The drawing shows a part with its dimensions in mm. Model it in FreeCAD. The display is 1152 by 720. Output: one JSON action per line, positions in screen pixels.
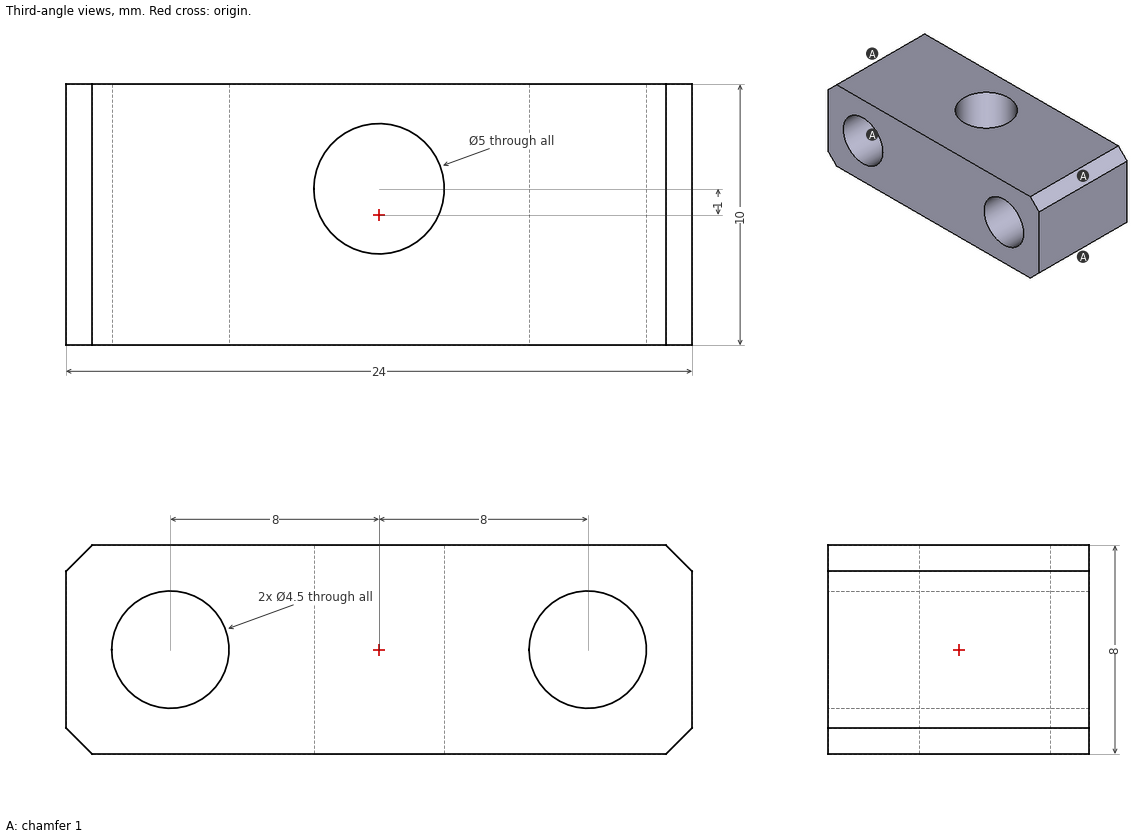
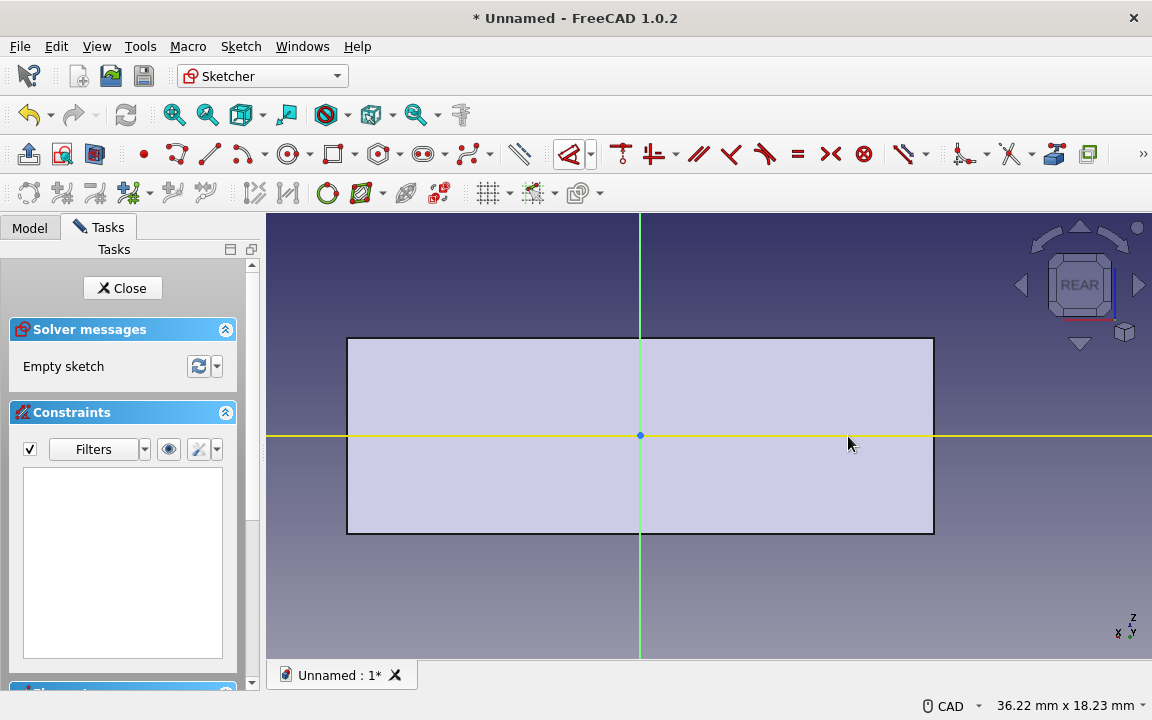
{"action": "left_click", "coordinate": [288, 154]}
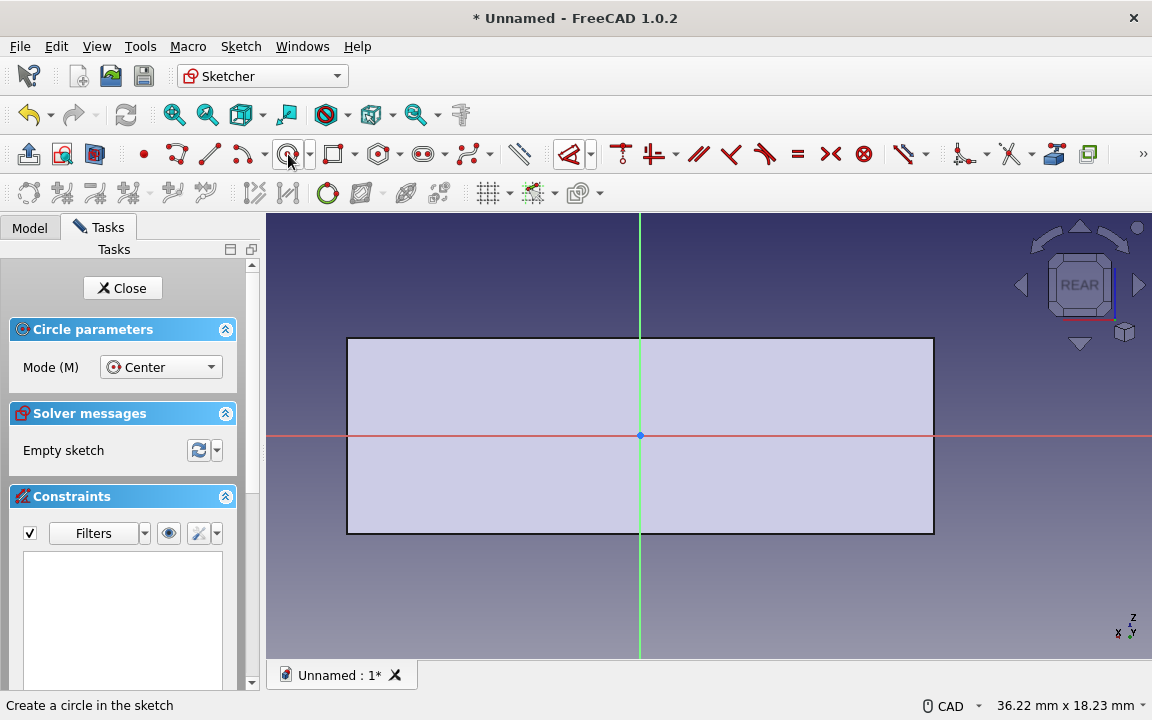
{"action": "left_click", "coordinate": [836, 436]}
{"action": "left_click", "coordinate": [875, 397]}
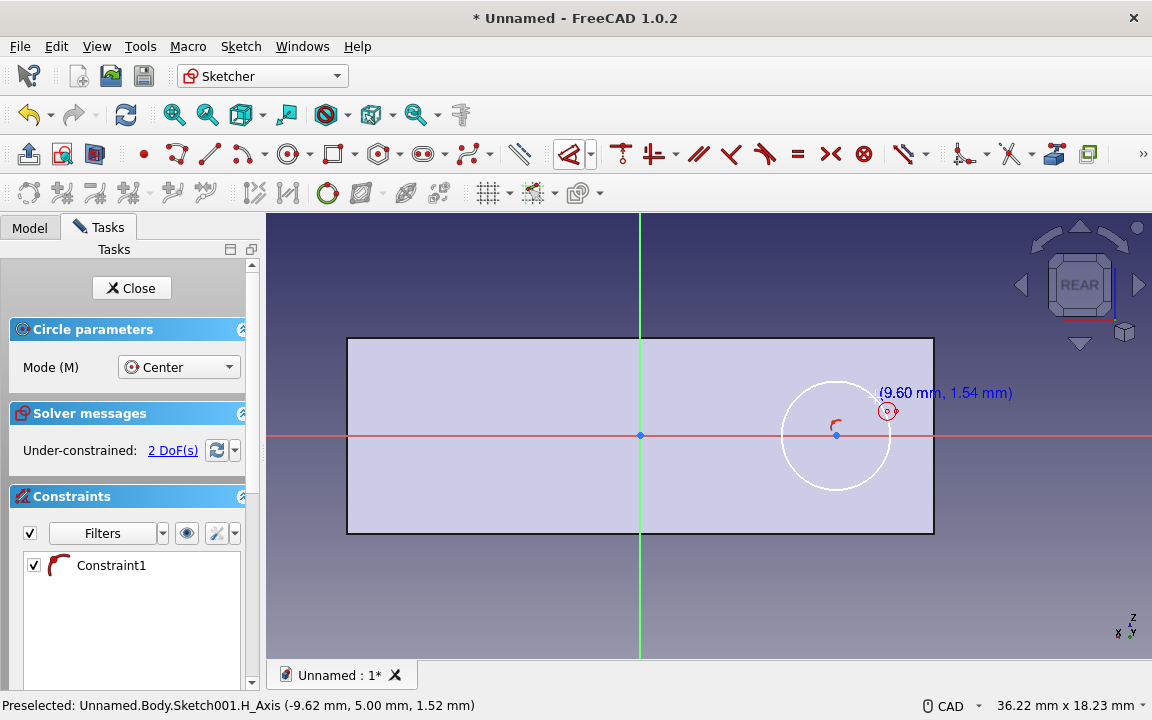
{"action": "left_click", "coordinate": [445, 436]}
{"action": "left_click", "coordinate": [484, 397]}
{"action": "key", "text": "Escape"}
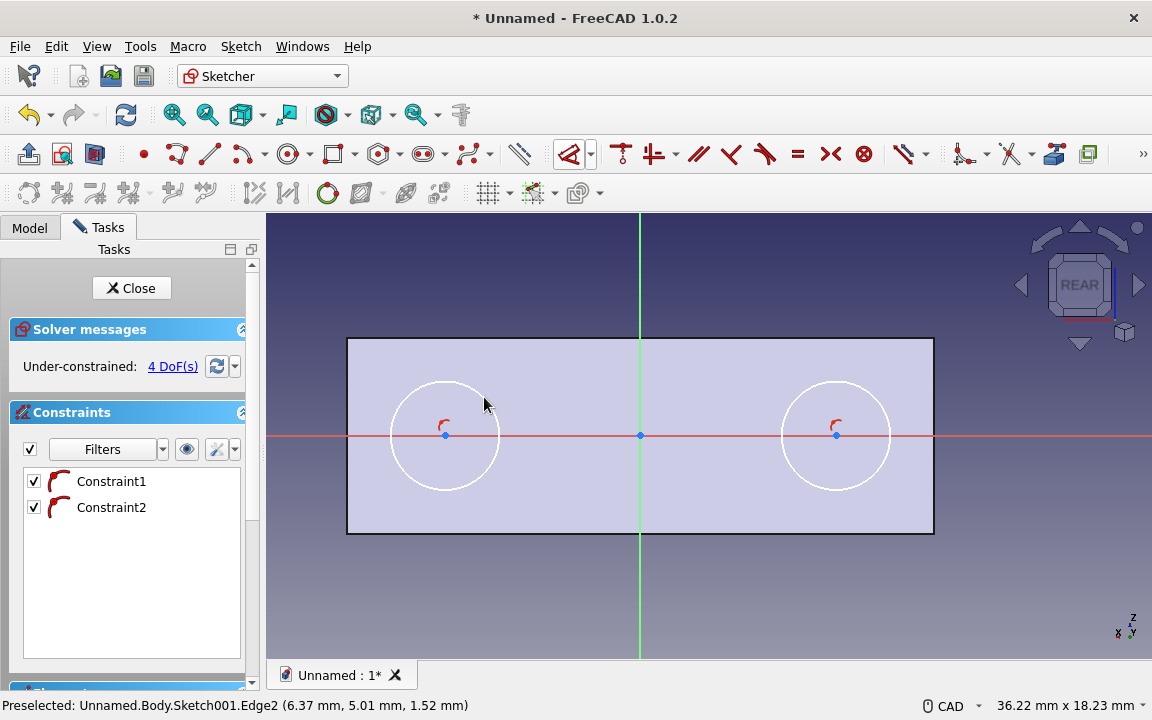
{"action": "left_click", "coordinate": [874, 397]}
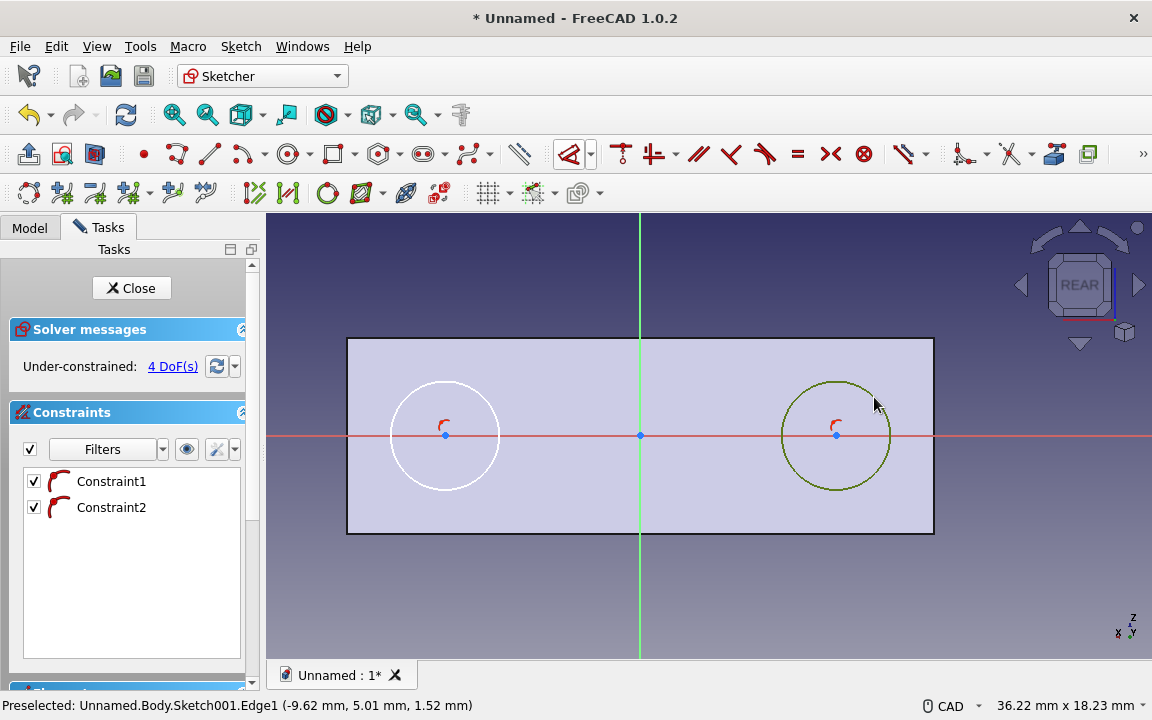
{"action": "left_click", "coordinate": [483, 397]}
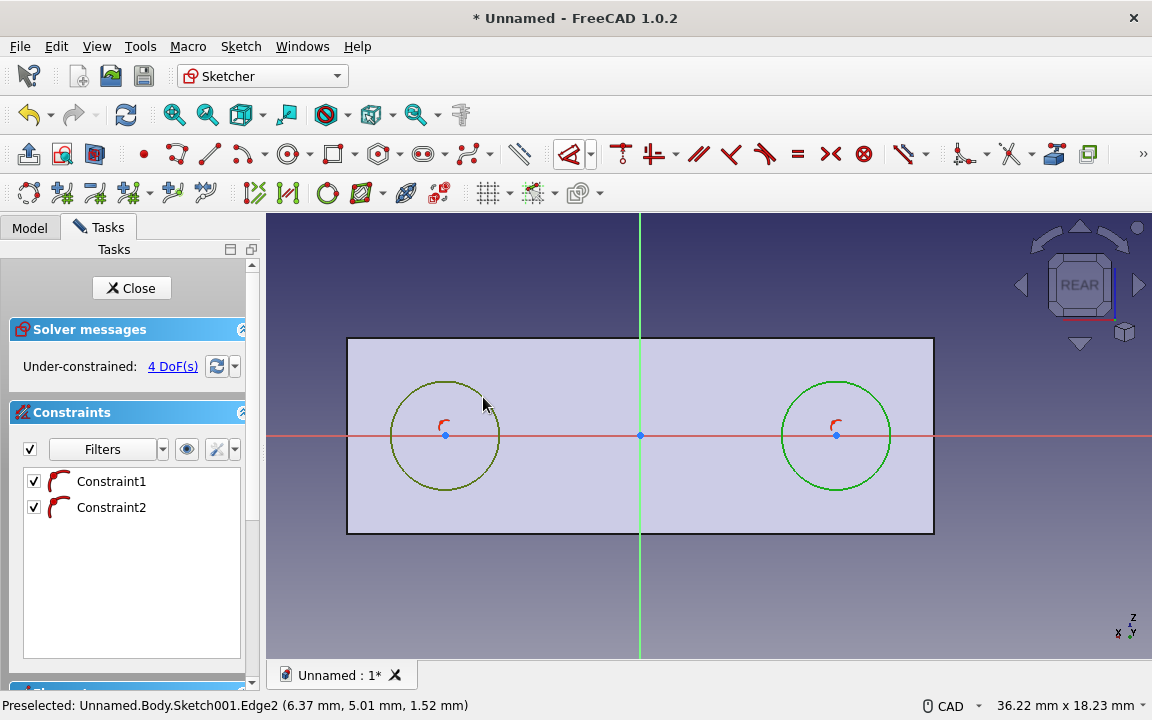
{"action": "left_click", "coordinate": [798, 154]}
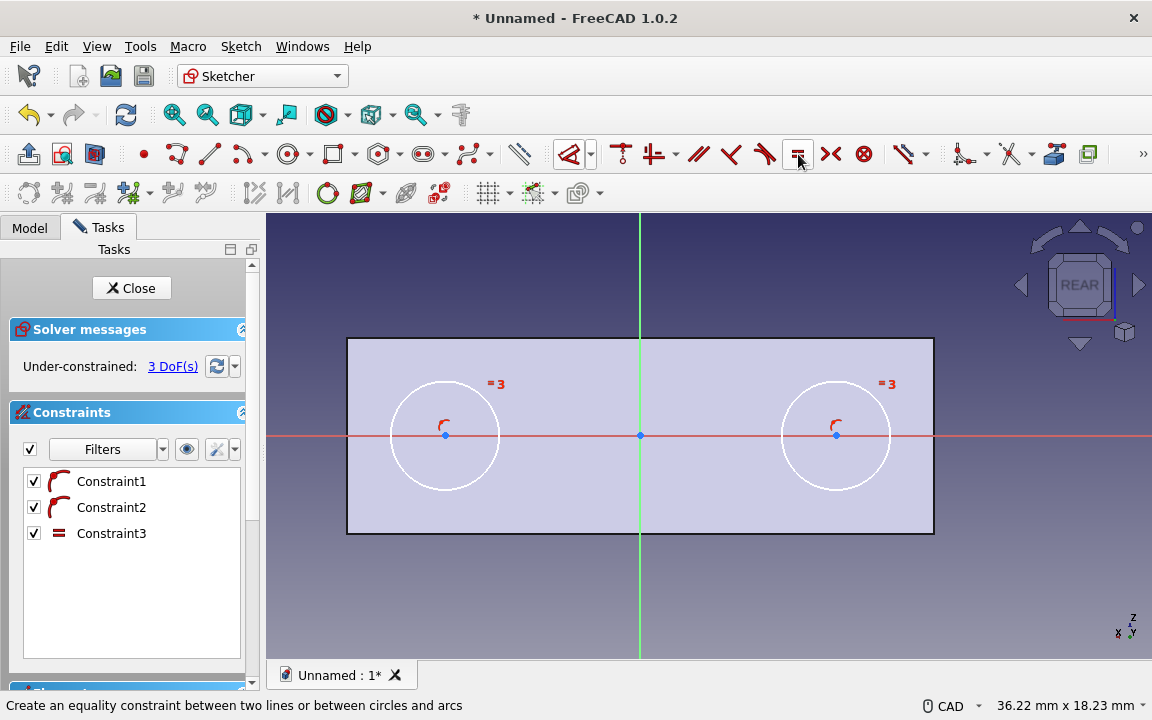
{"action": "left_click", "coordinate": [874, 397]}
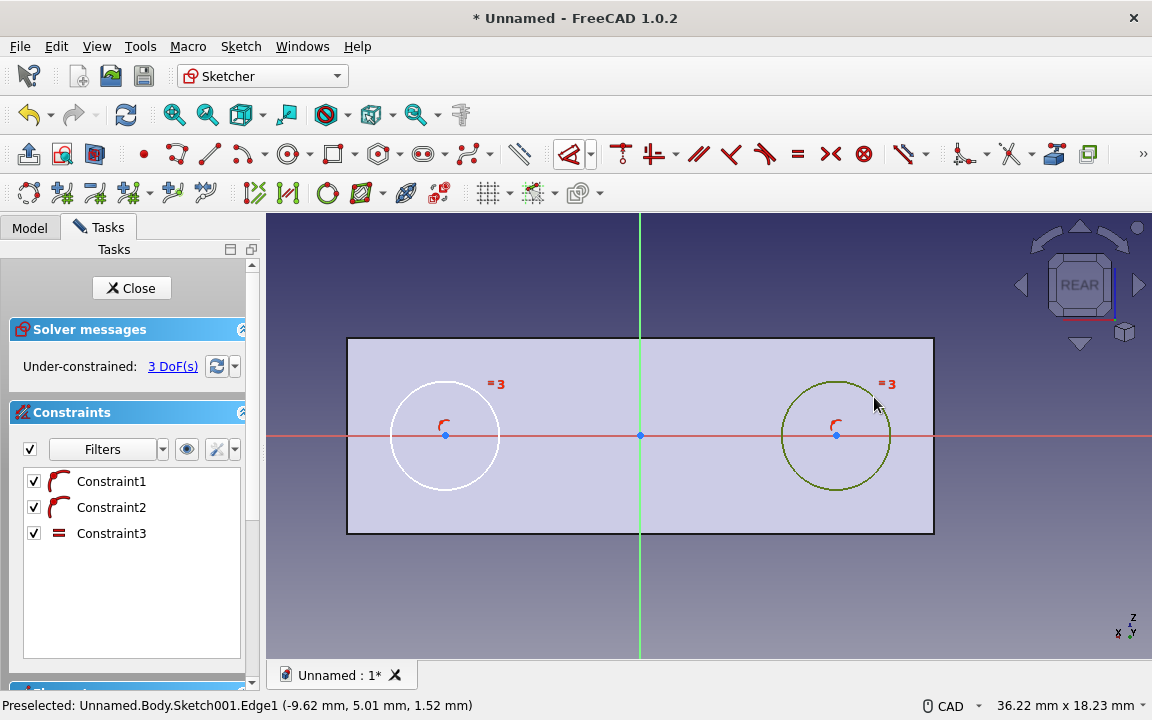
{"action": "key", "text": "k o"}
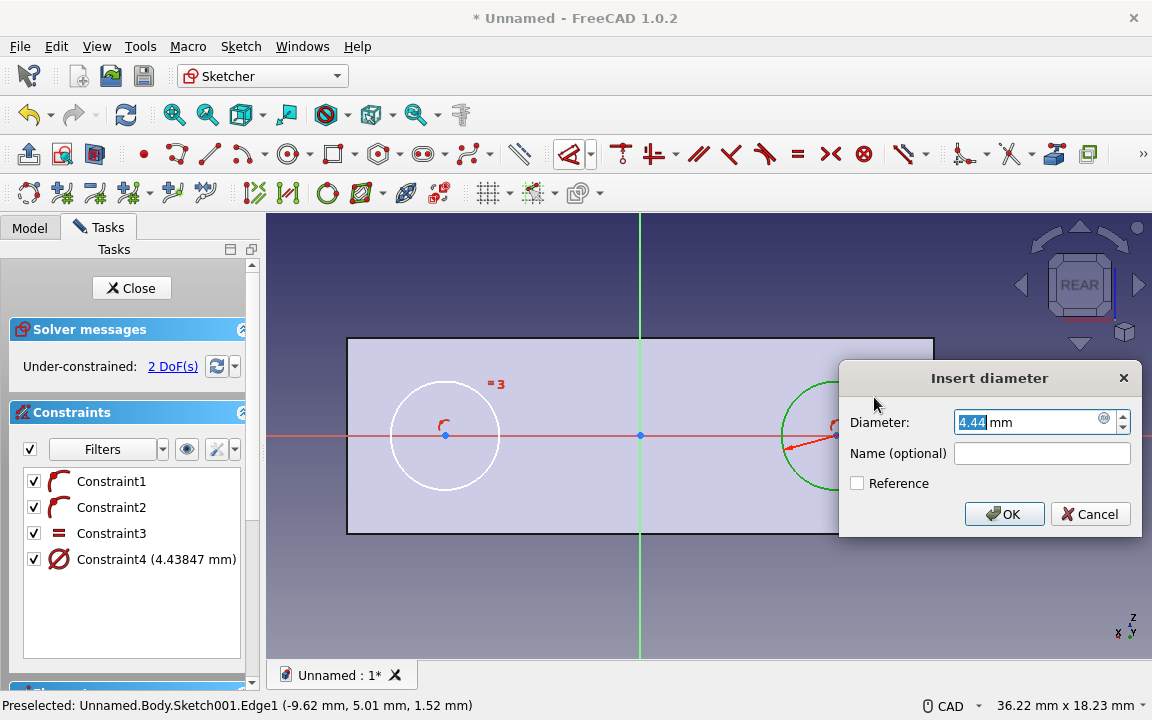
{"action": "type", "text": "4.5"}
{"action": "key", "text": "Return"}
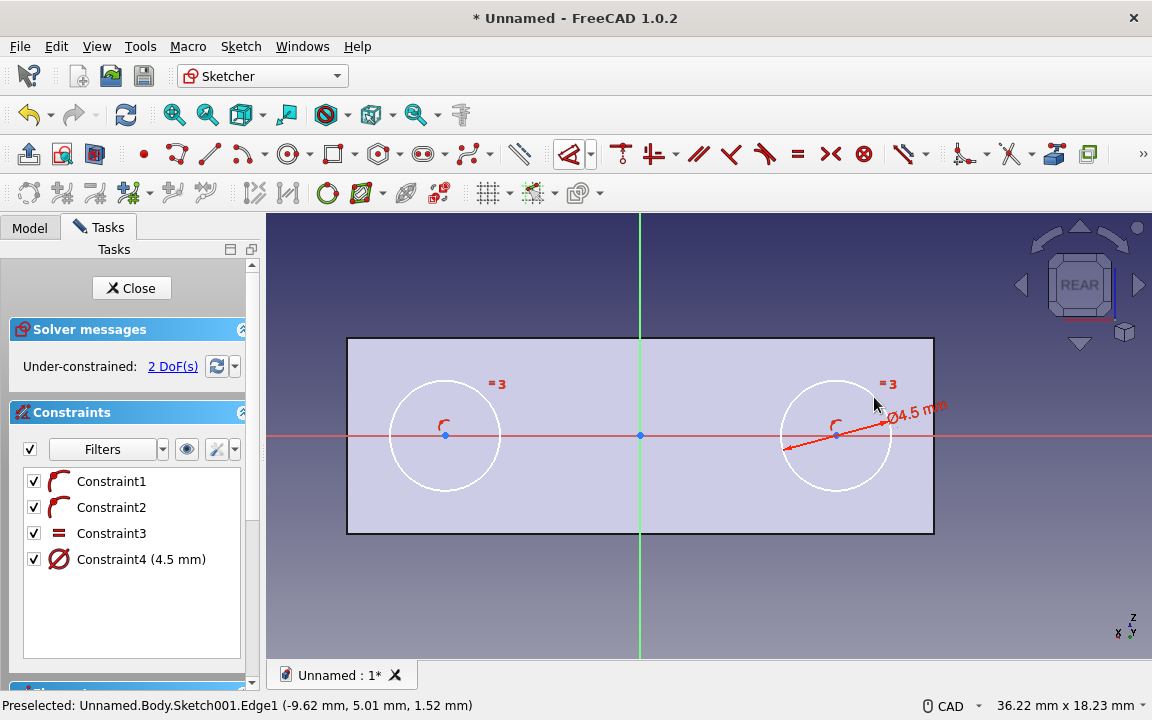
{"action": "left_click", "coordinate": [836, 436]}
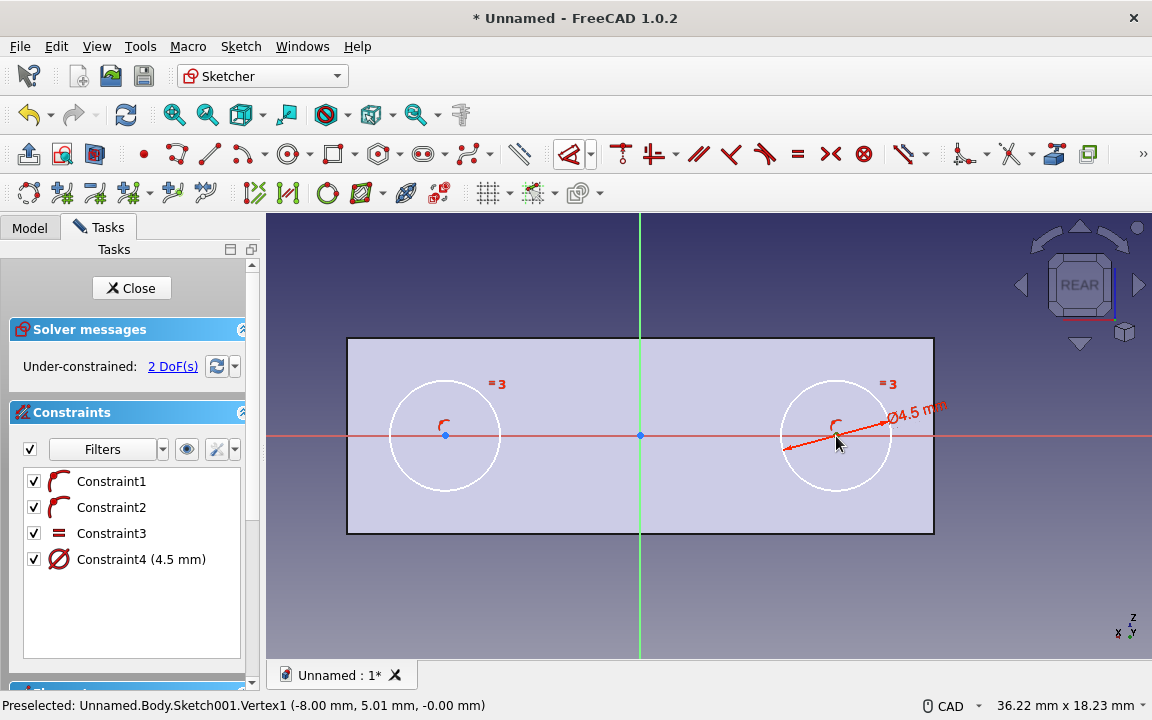
{"action": "key", "text": "l"}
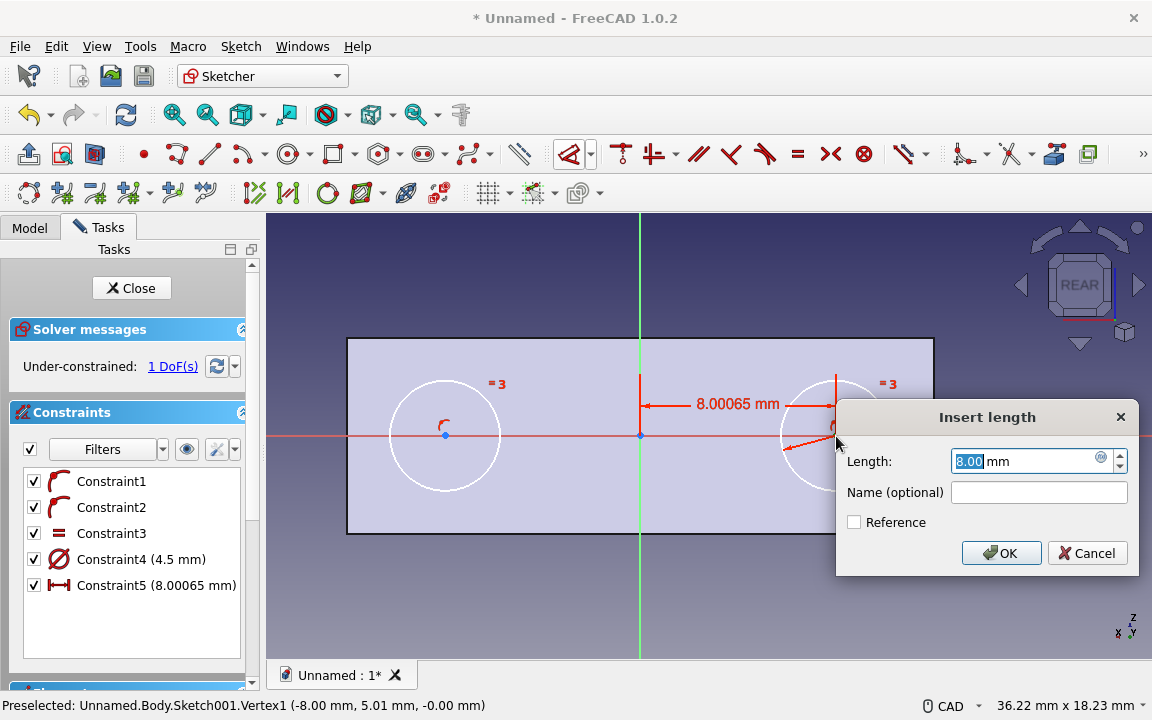
{"action": "type", "text": "8"}
{"action": "key", "text": "Return"}